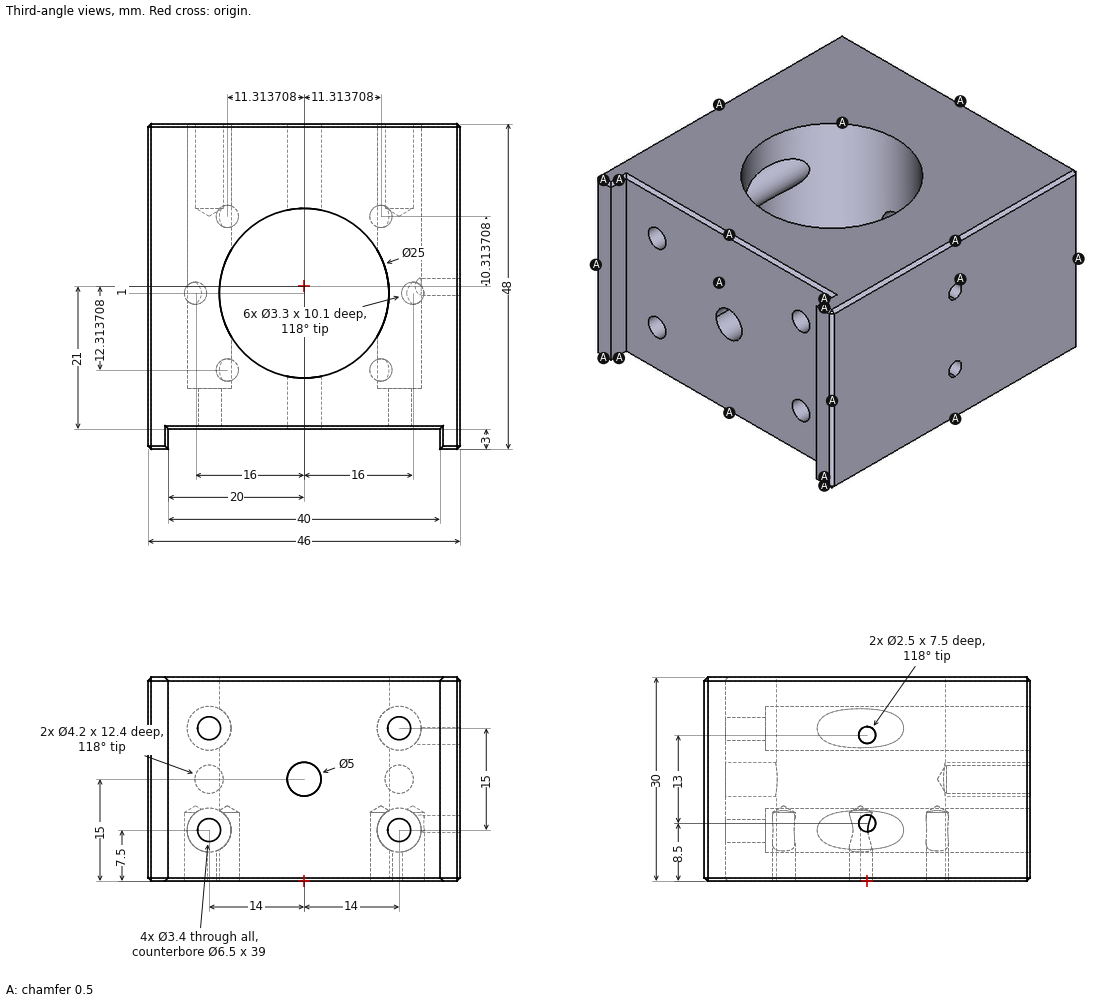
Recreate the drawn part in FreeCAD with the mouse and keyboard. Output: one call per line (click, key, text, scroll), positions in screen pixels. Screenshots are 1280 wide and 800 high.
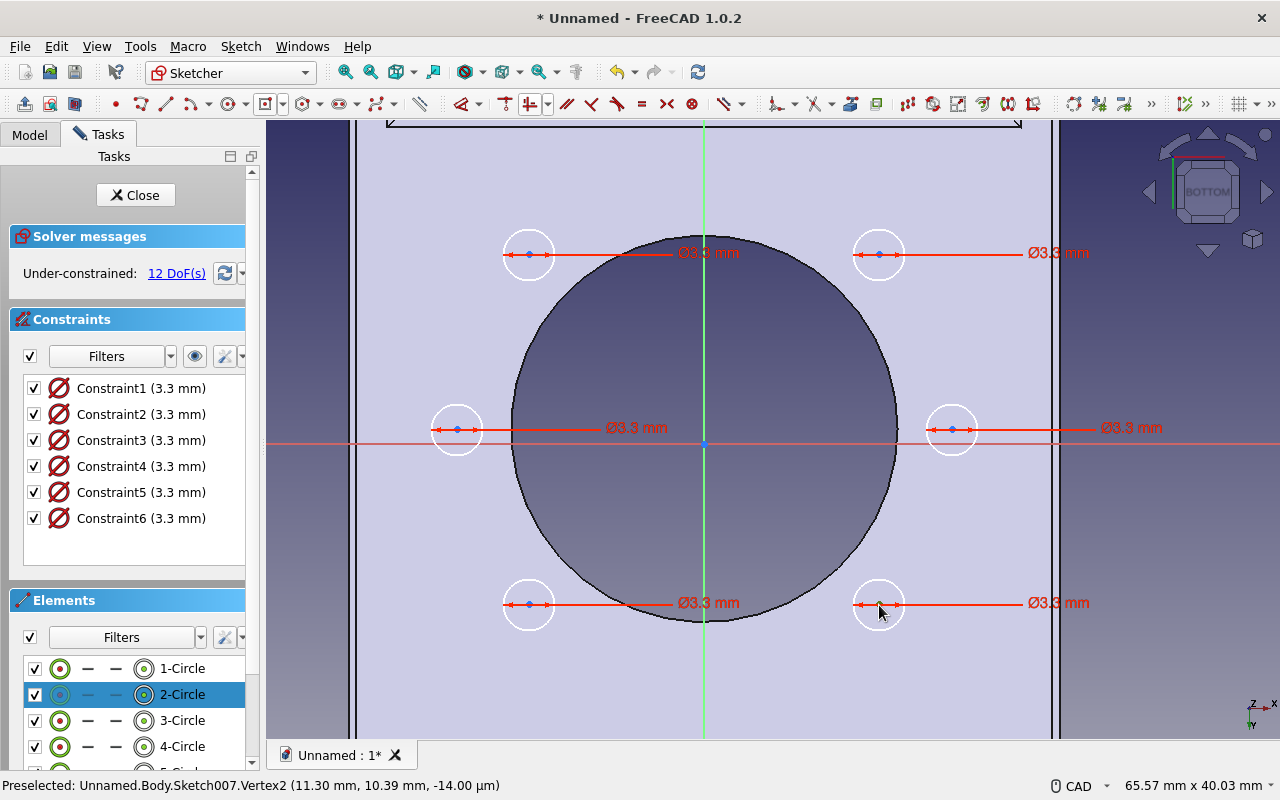
click(529, 605)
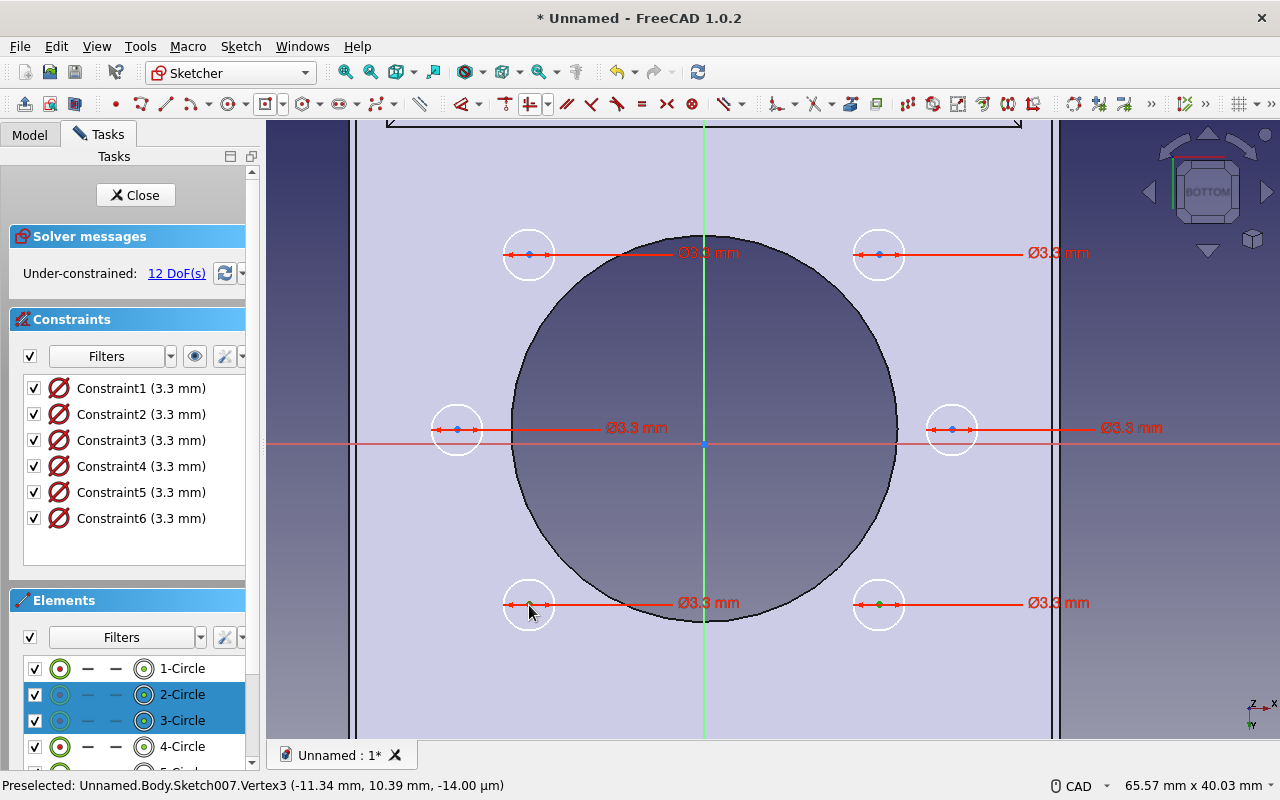
key(h)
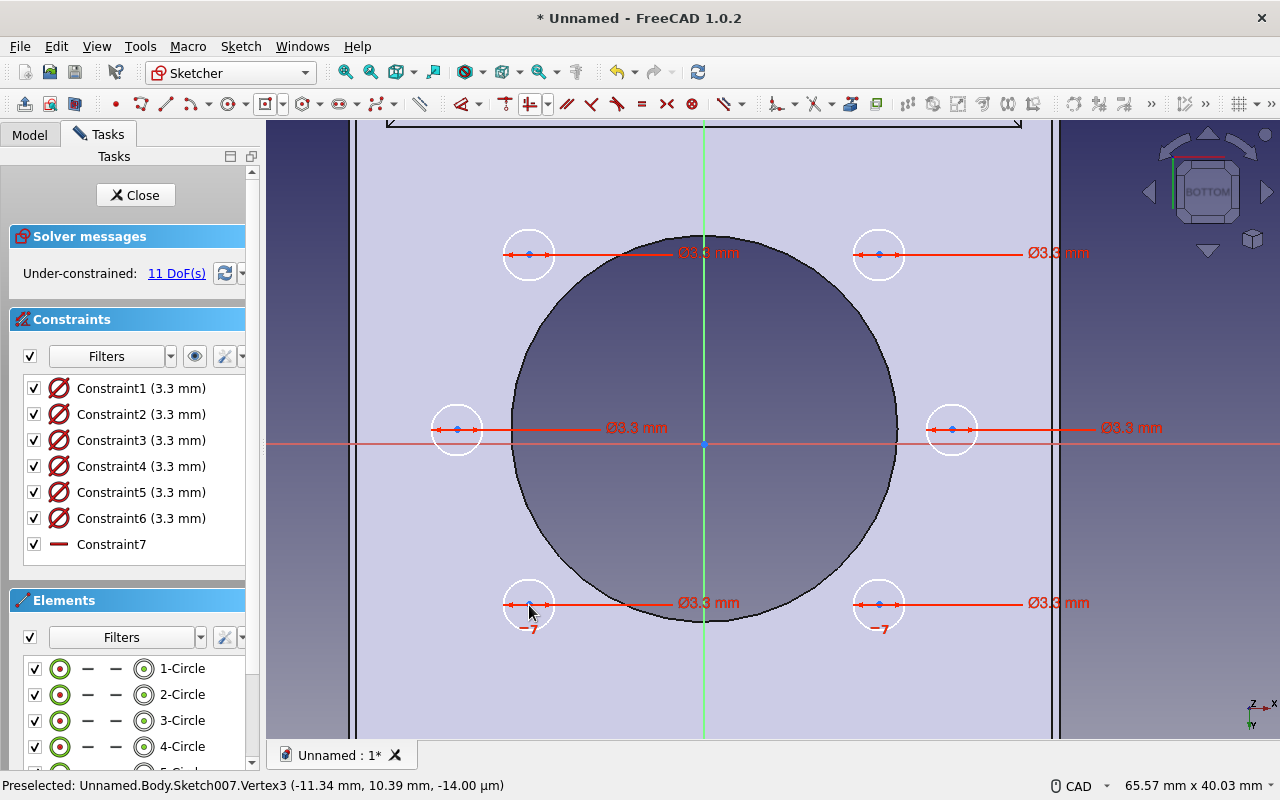
click(952, 430)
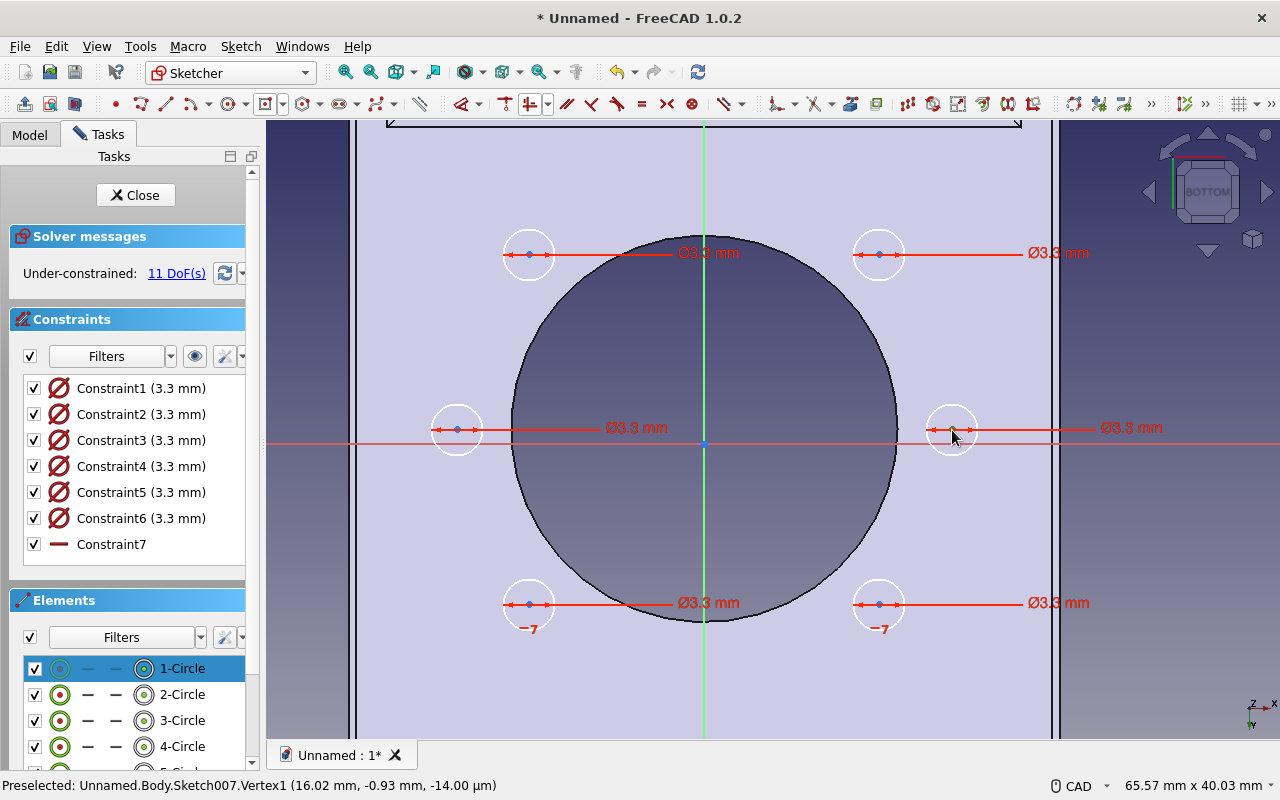
click(457, 430)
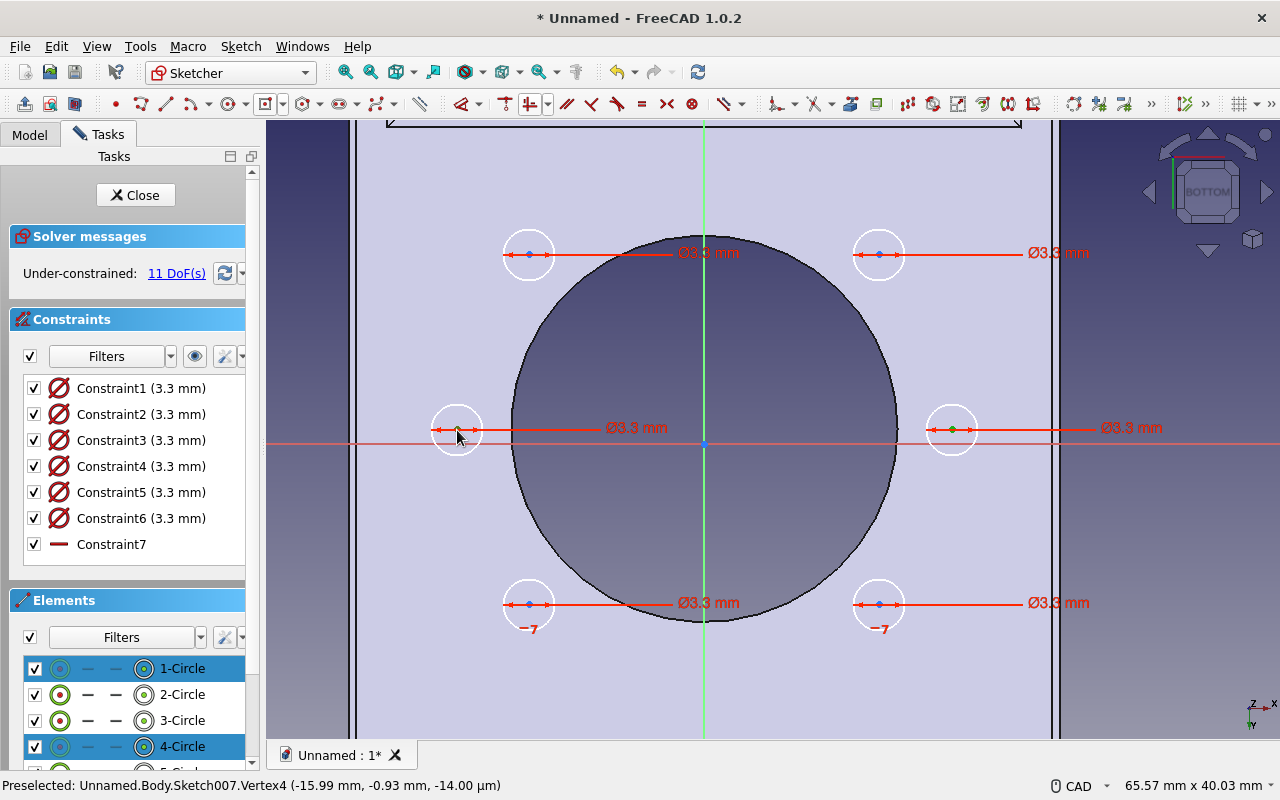
key(h)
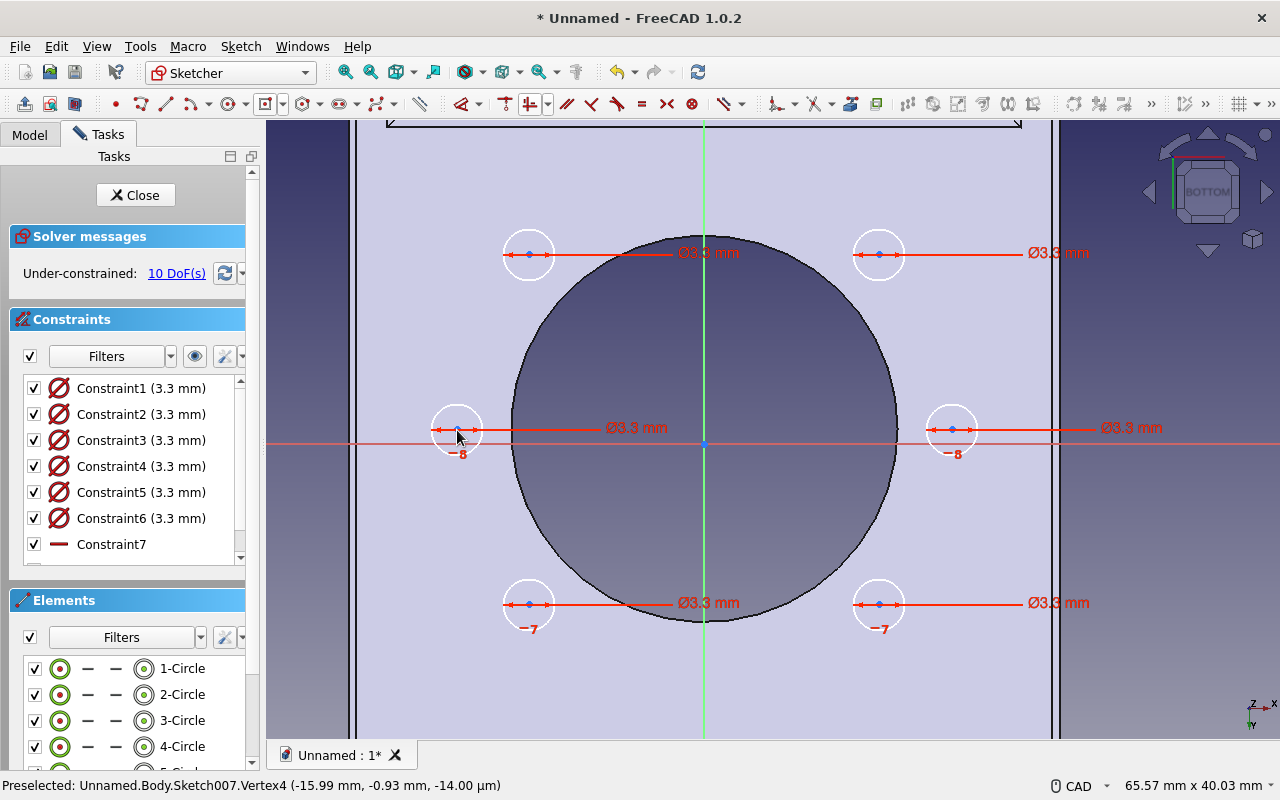
click(529, 605)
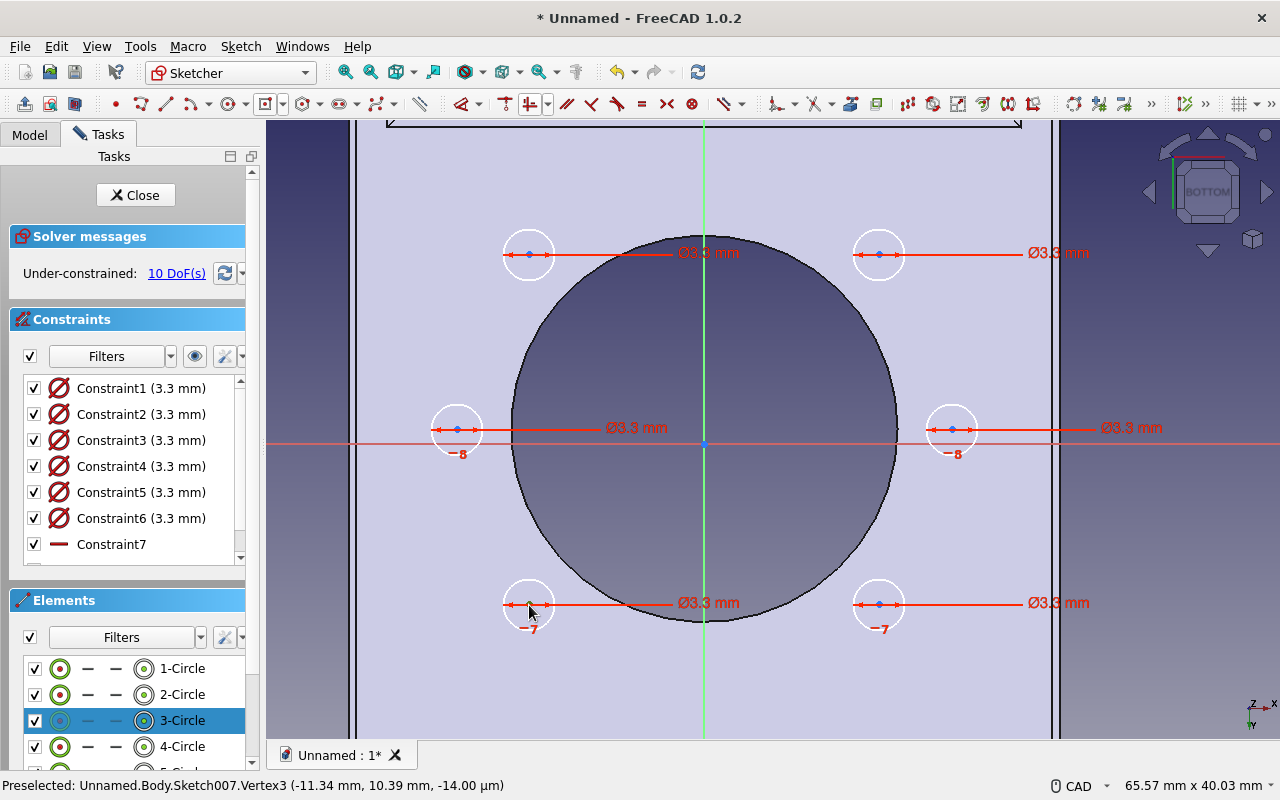
click(529, 255)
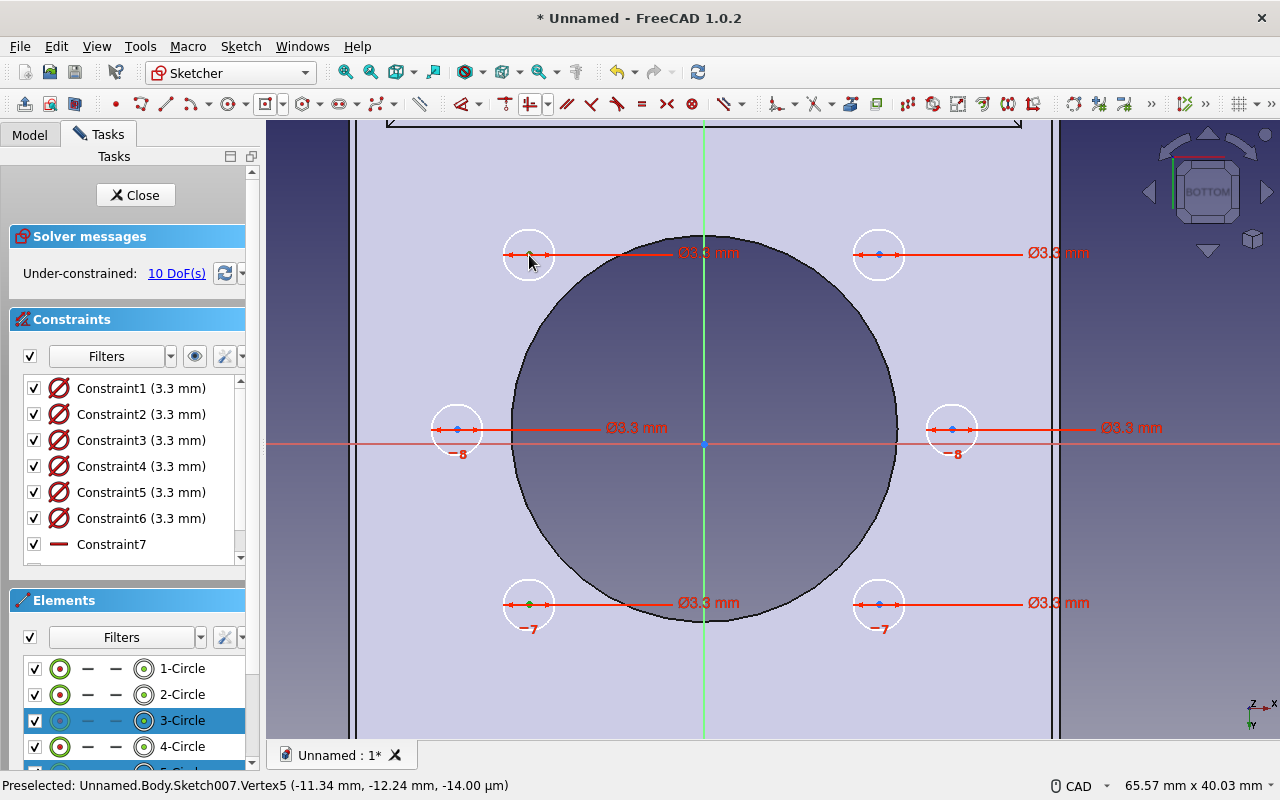
key(v)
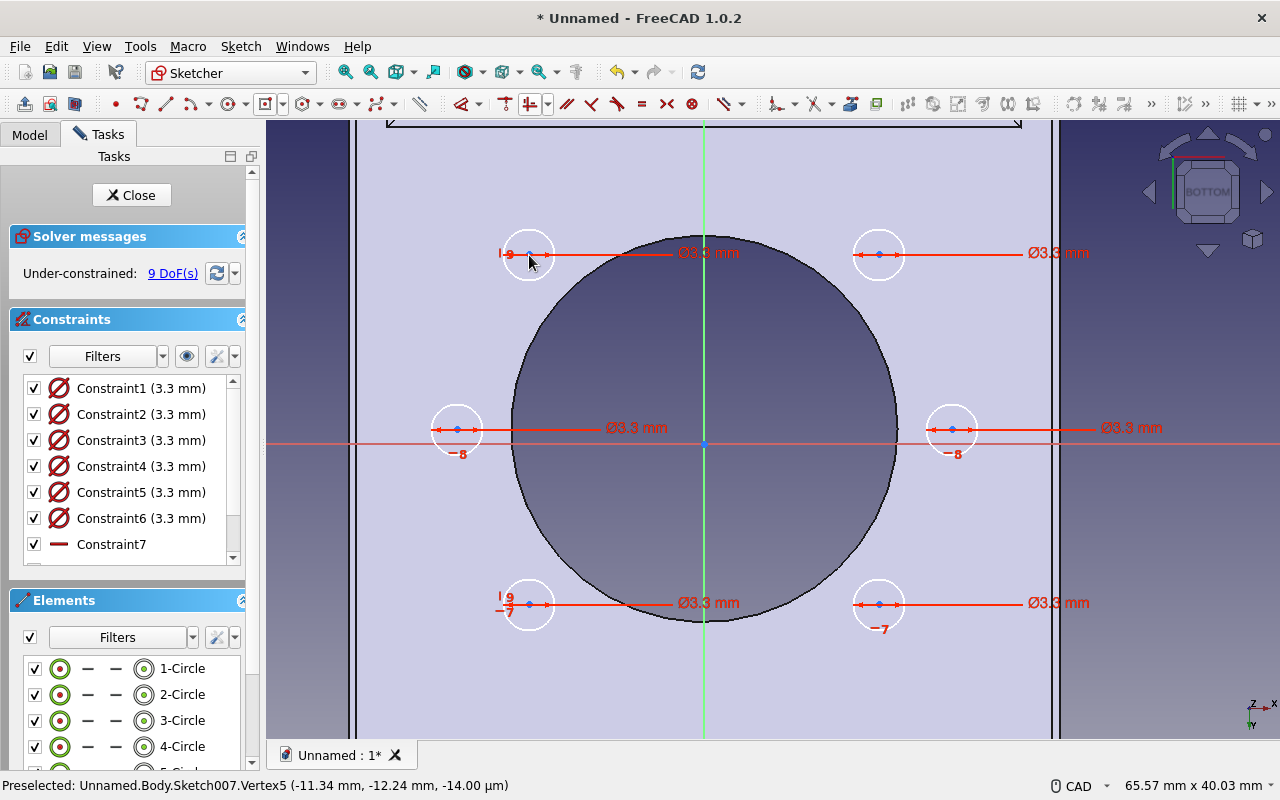
click(879, 605)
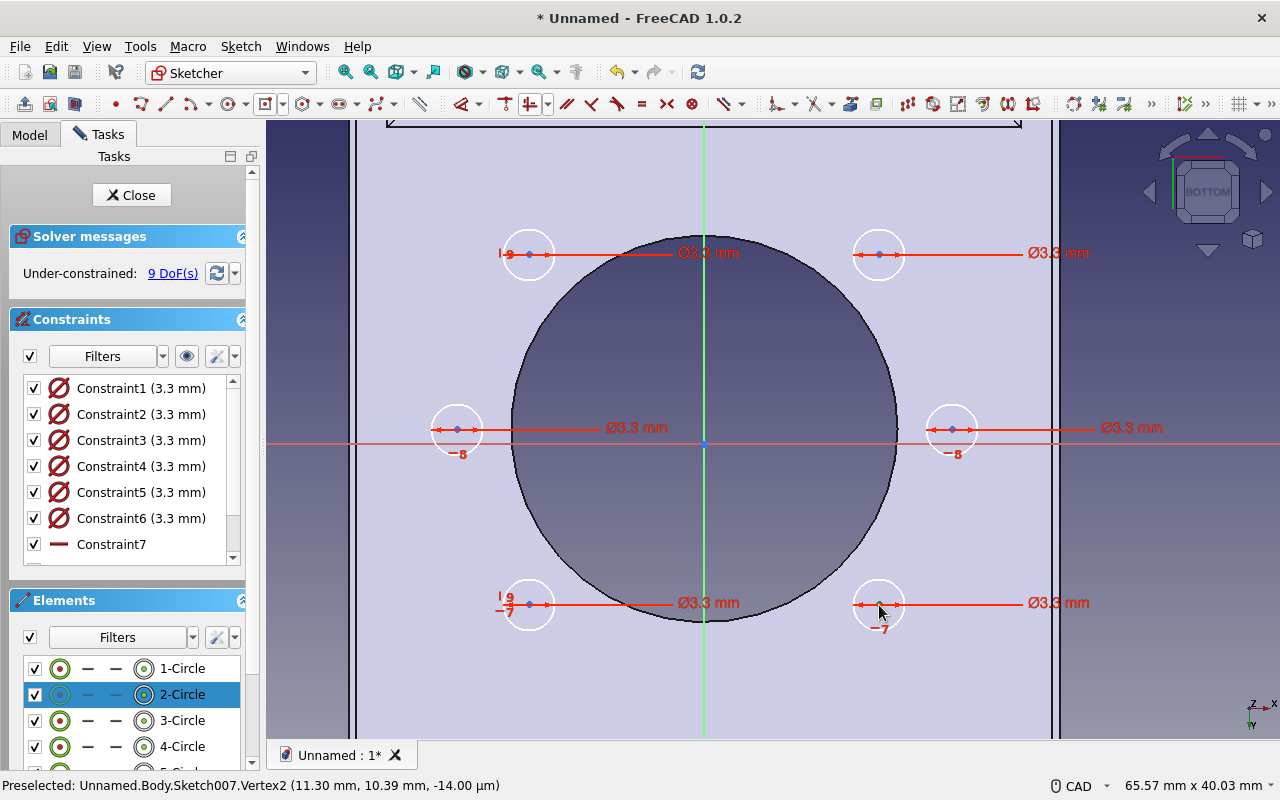
click(879, 255)